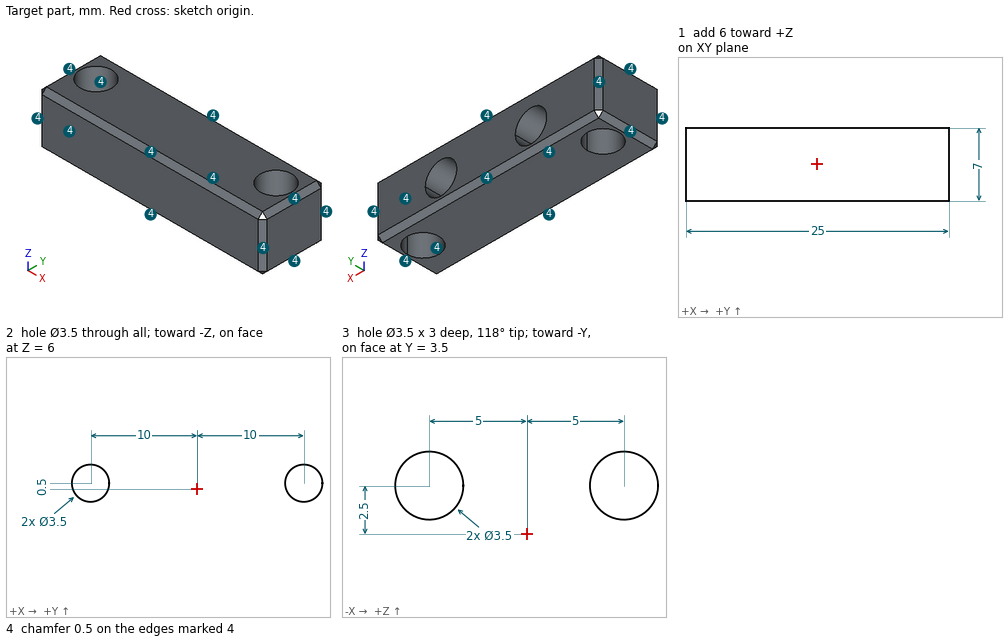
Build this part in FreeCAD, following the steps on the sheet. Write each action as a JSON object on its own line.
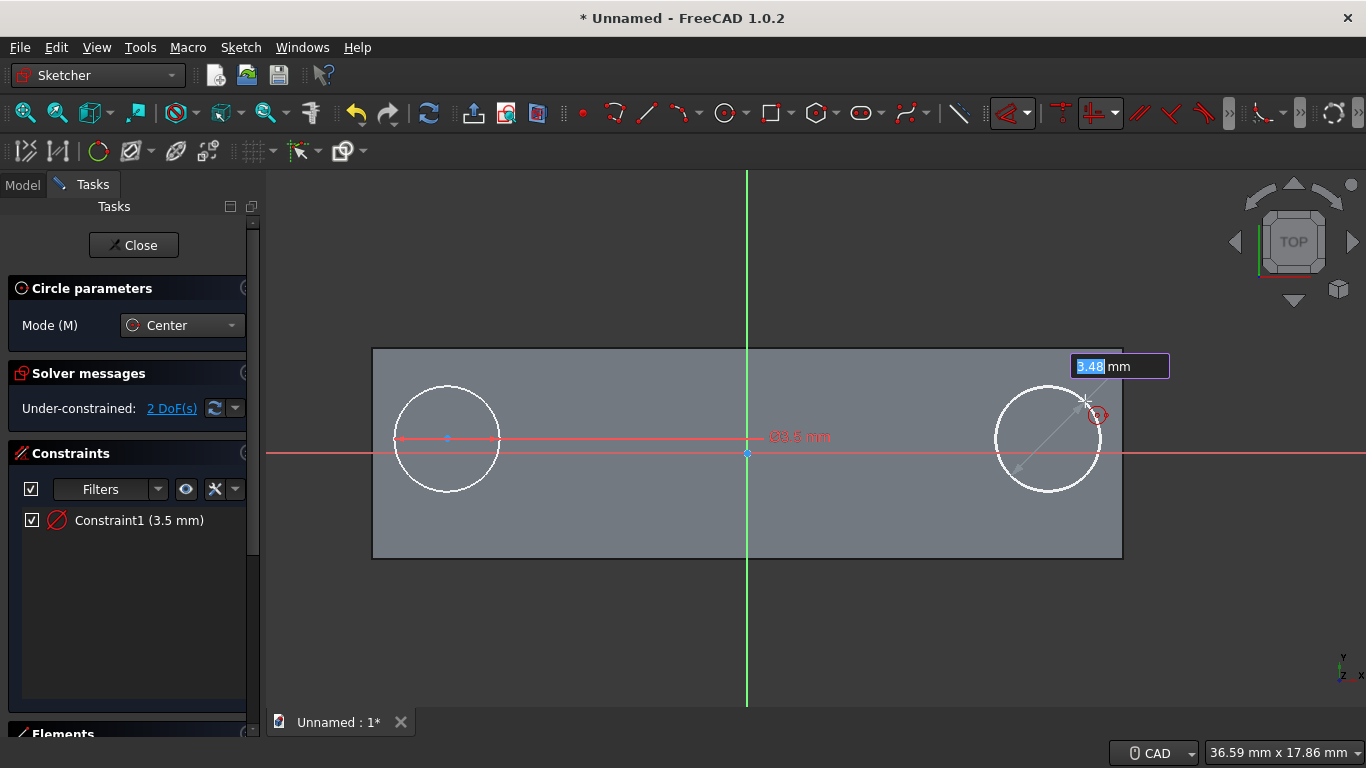
{"action": "type", "text": "3.5"}
{"action": "key", "text": "Return"}
{"action": "key", "text": "Escape"}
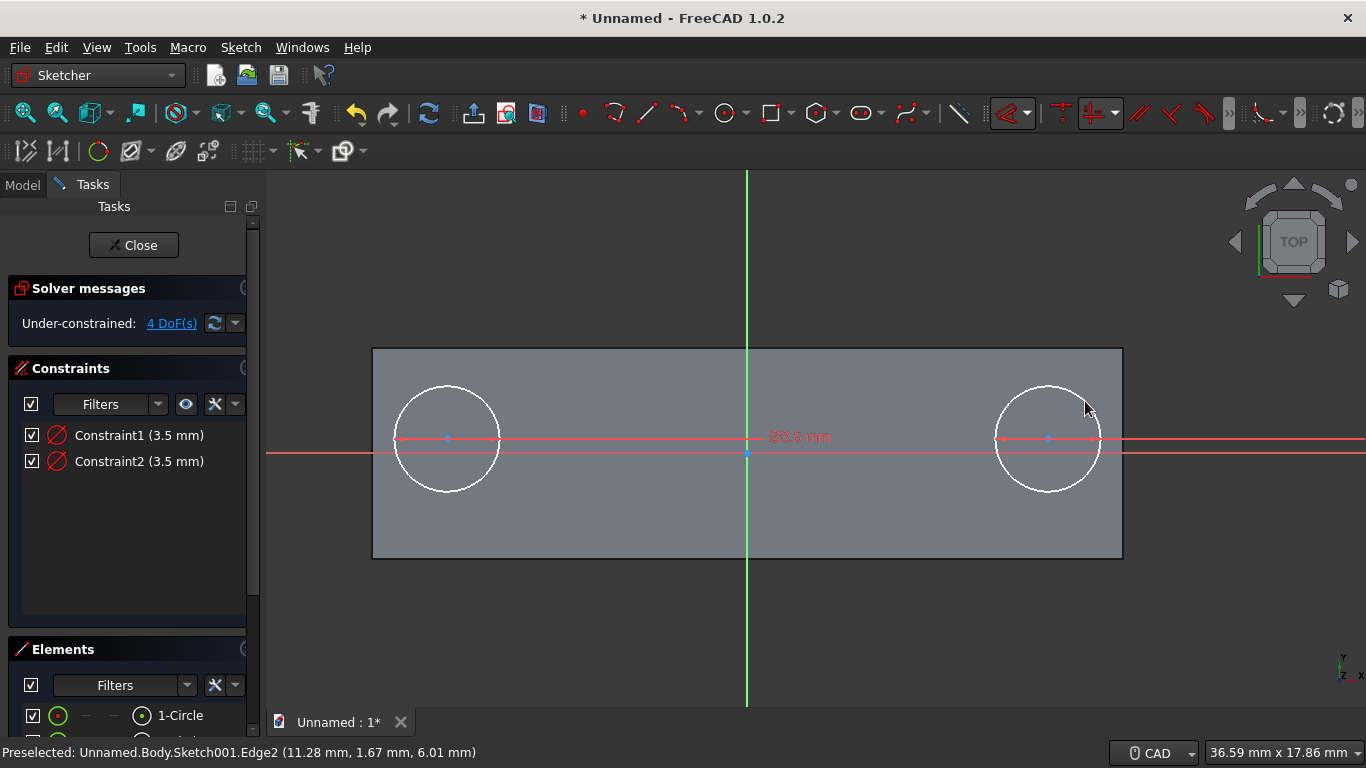
{"action": "left_click", "coordinate": [447, 439]}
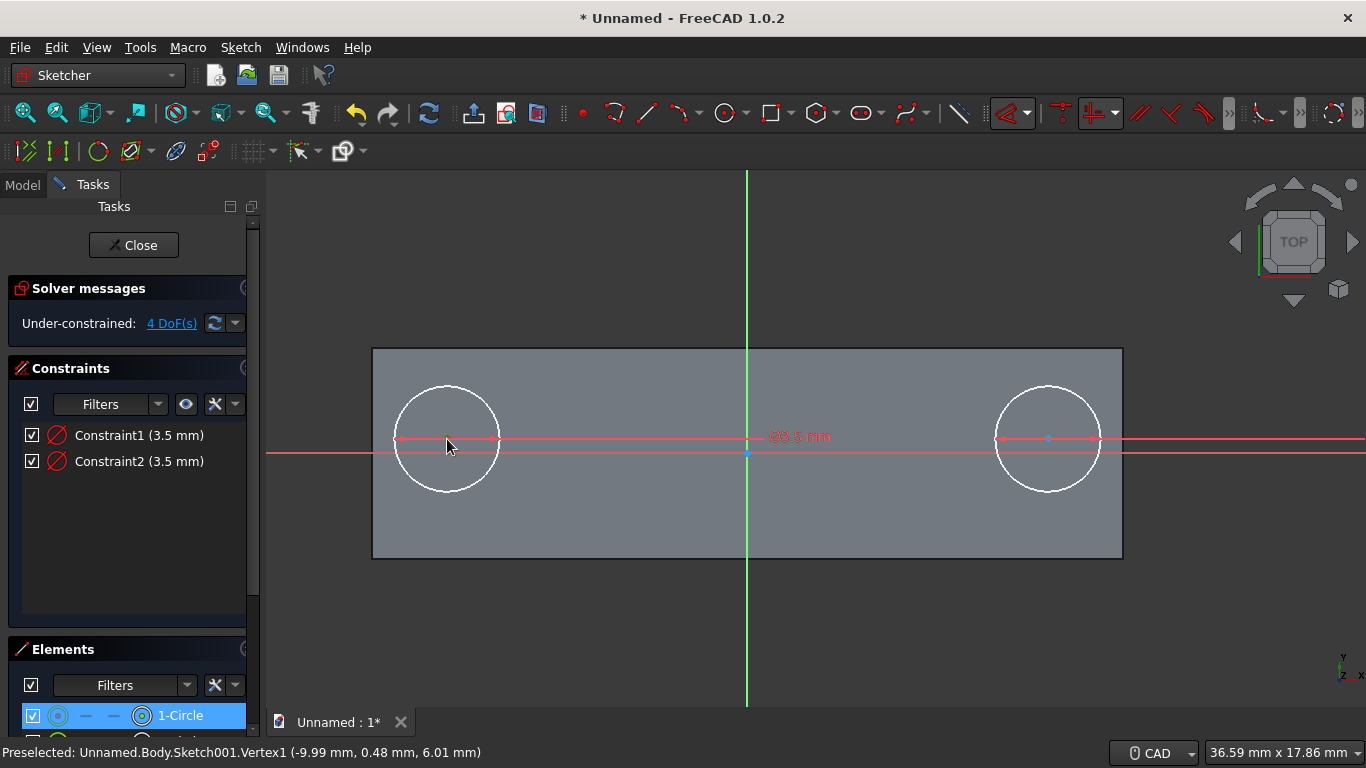
{"action": "left_click", "coordinate": [1048, 439]}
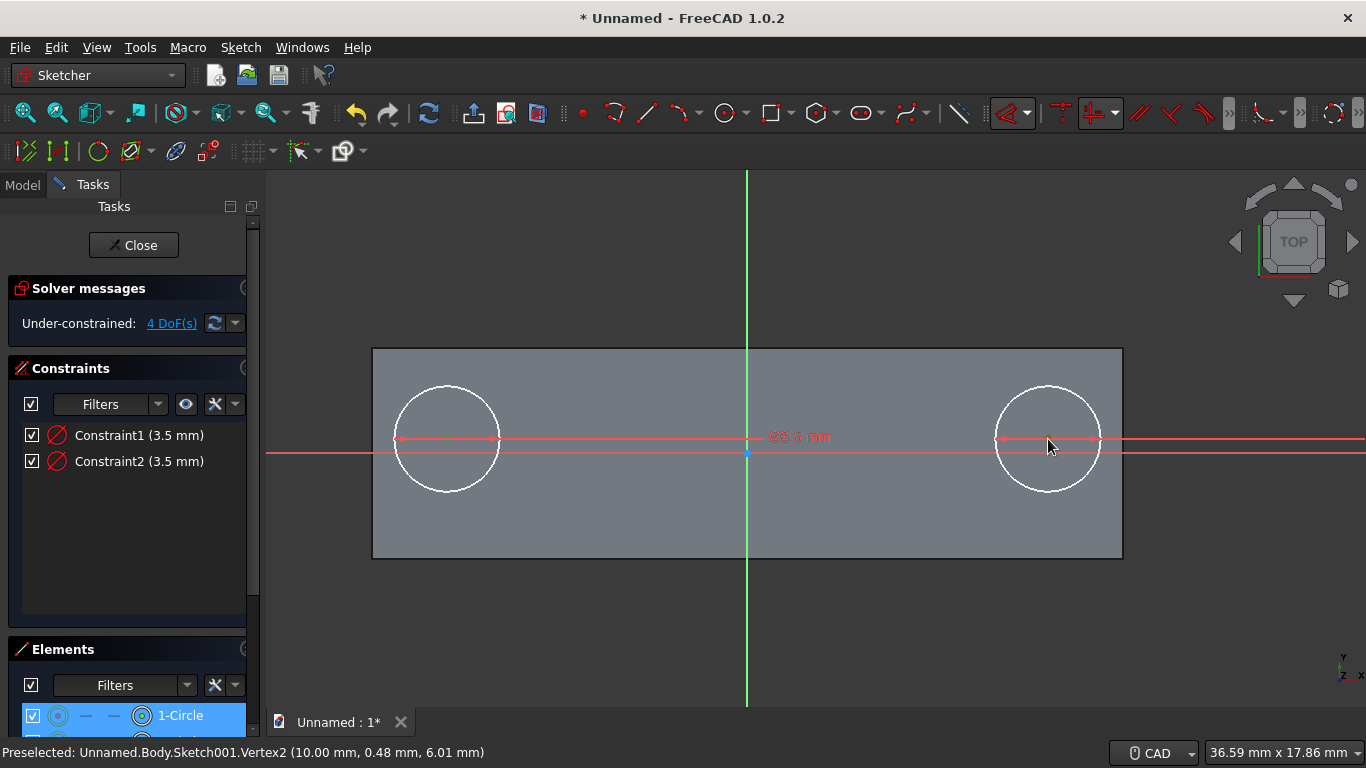
{"action": "left_click", "coordinate": [1118, 114]}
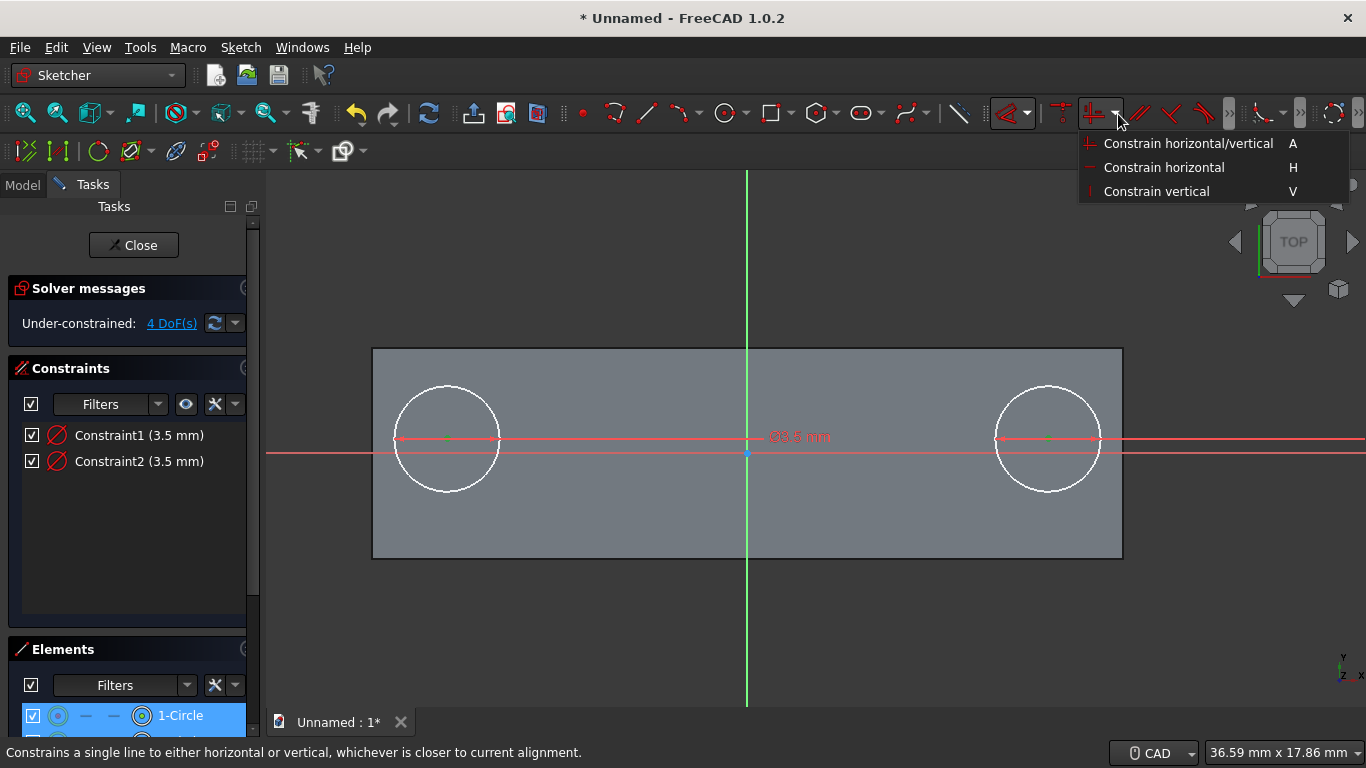
{"action": "left_click", "coordinate": [1214, 167]}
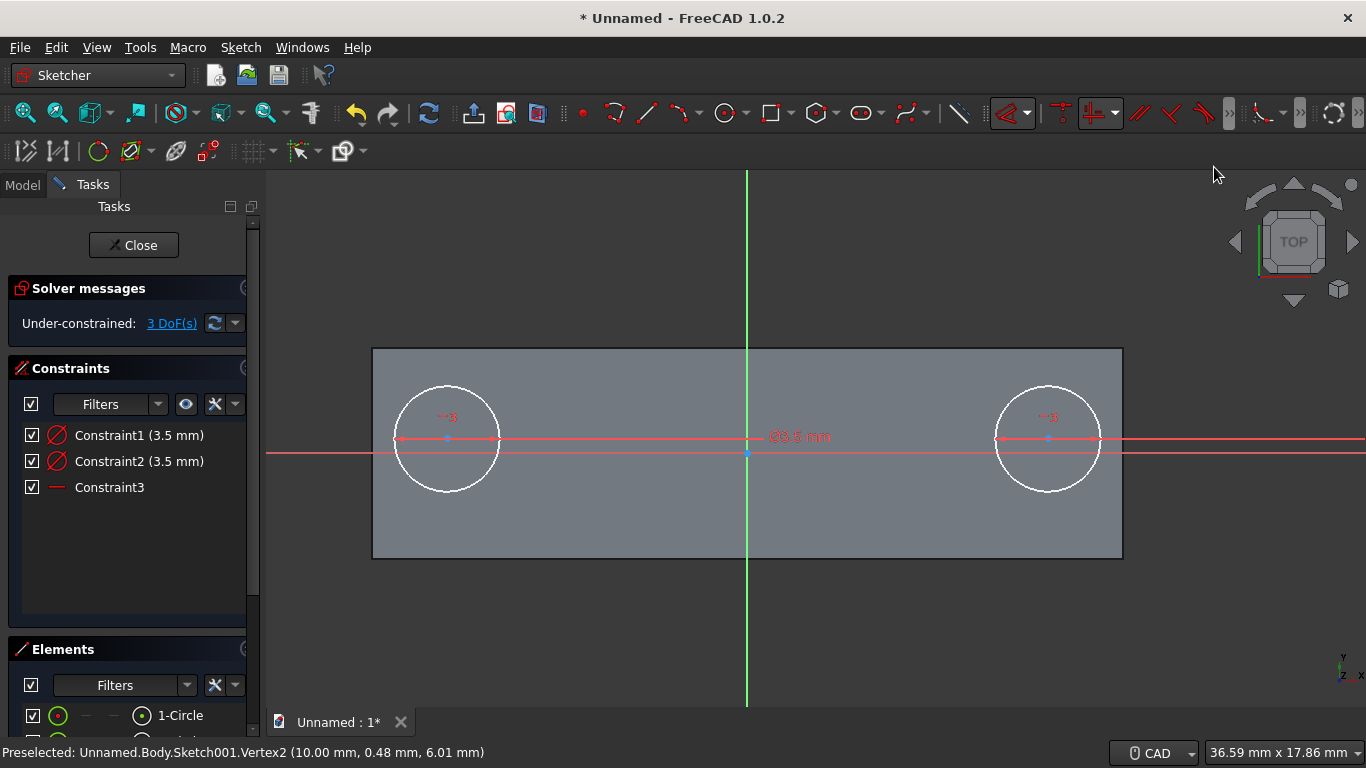
{"action": "left_click", "coordinate": [1006, 114]}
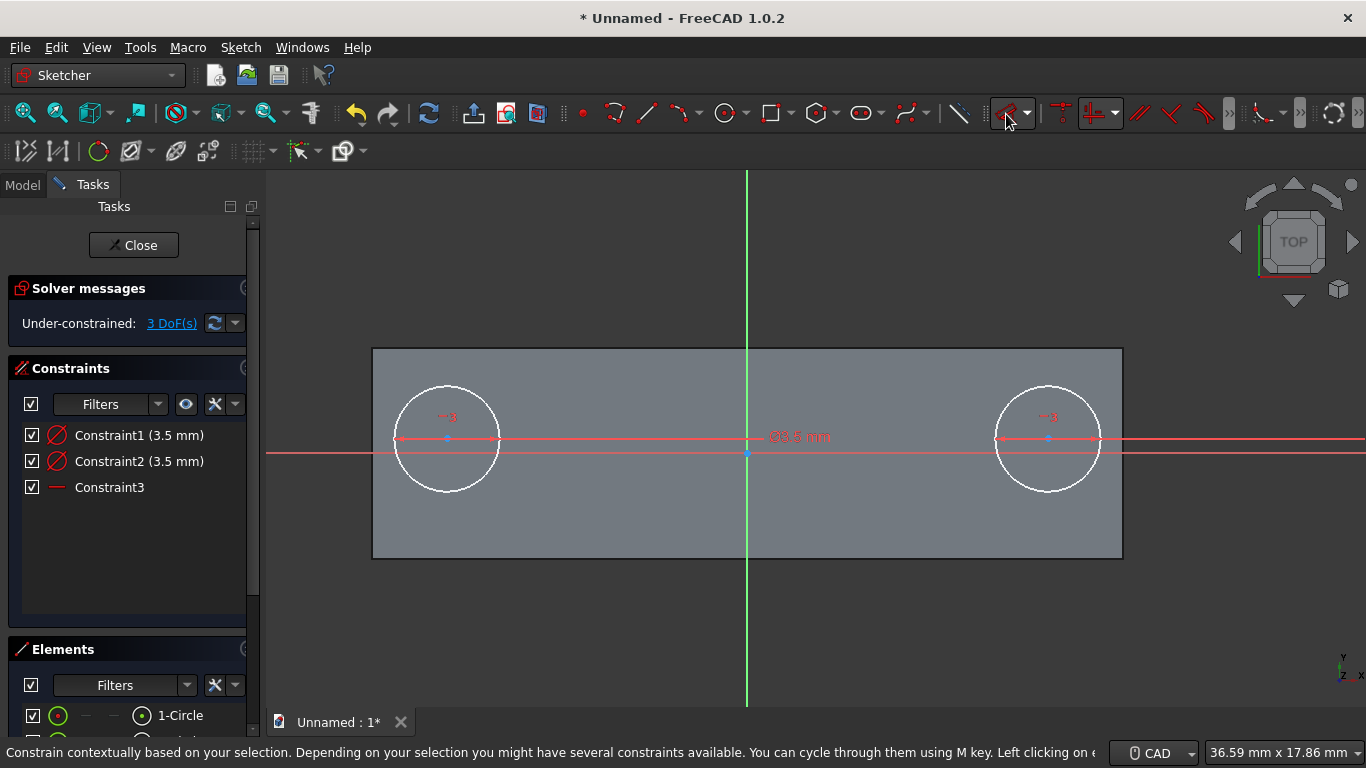
{"action": "left_click", "coordinate": [447, 439]}
{"action": "left_click", "coordinate": [597, 487]}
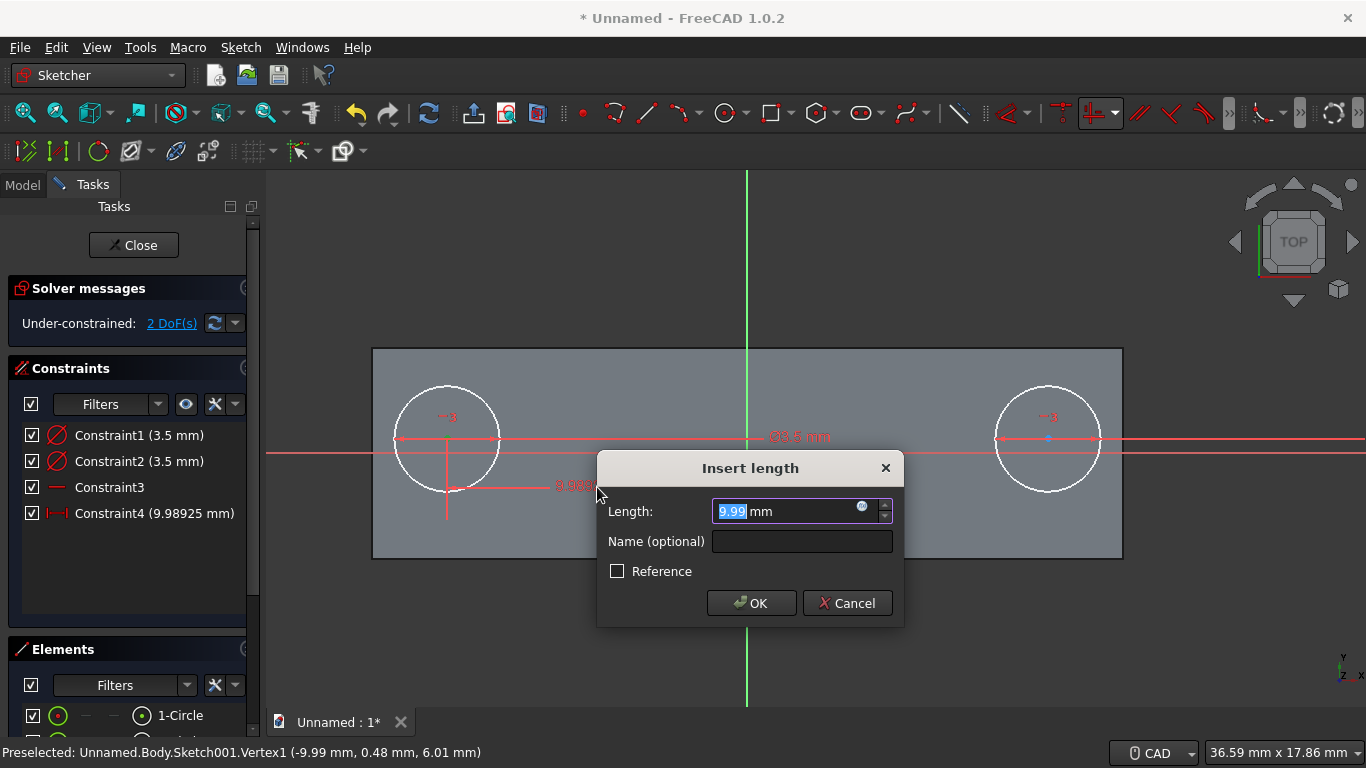
{"action": "type", "text": "10"}
{"action": "key", "text": "Return"}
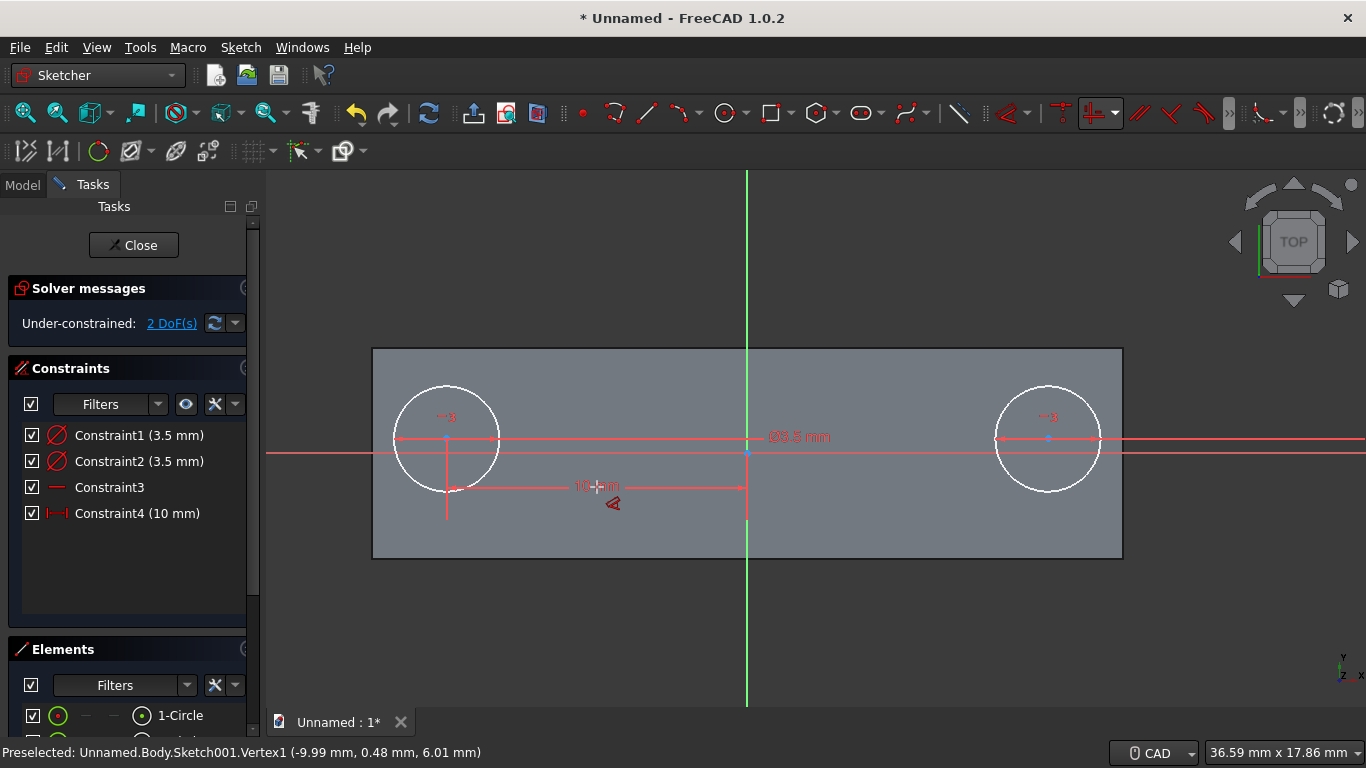
{"action": "left_click", "coordinate": [1048, 439]}
{"action": "left_click", "coordinate": [898, 487]}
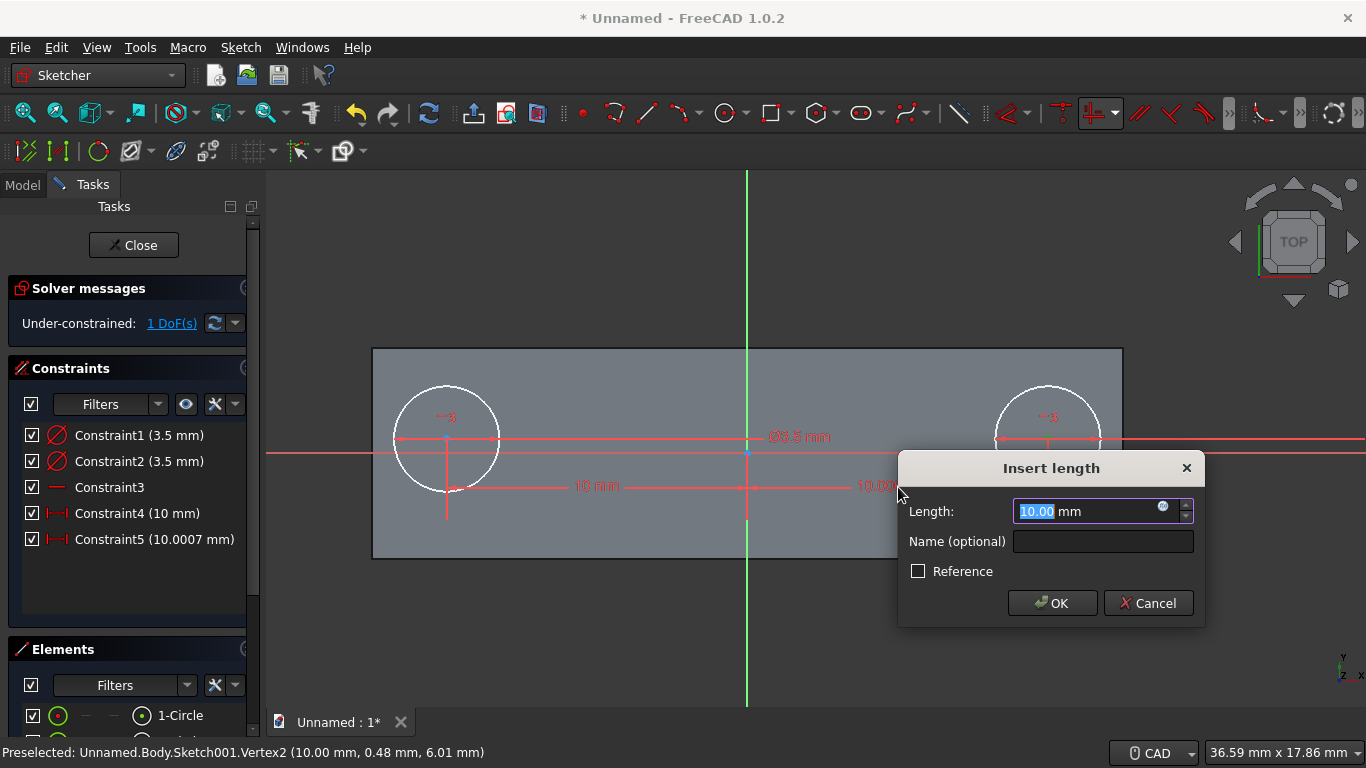
{"action": "type", "text": "10"}
{"action": "key", "text": "Return"}